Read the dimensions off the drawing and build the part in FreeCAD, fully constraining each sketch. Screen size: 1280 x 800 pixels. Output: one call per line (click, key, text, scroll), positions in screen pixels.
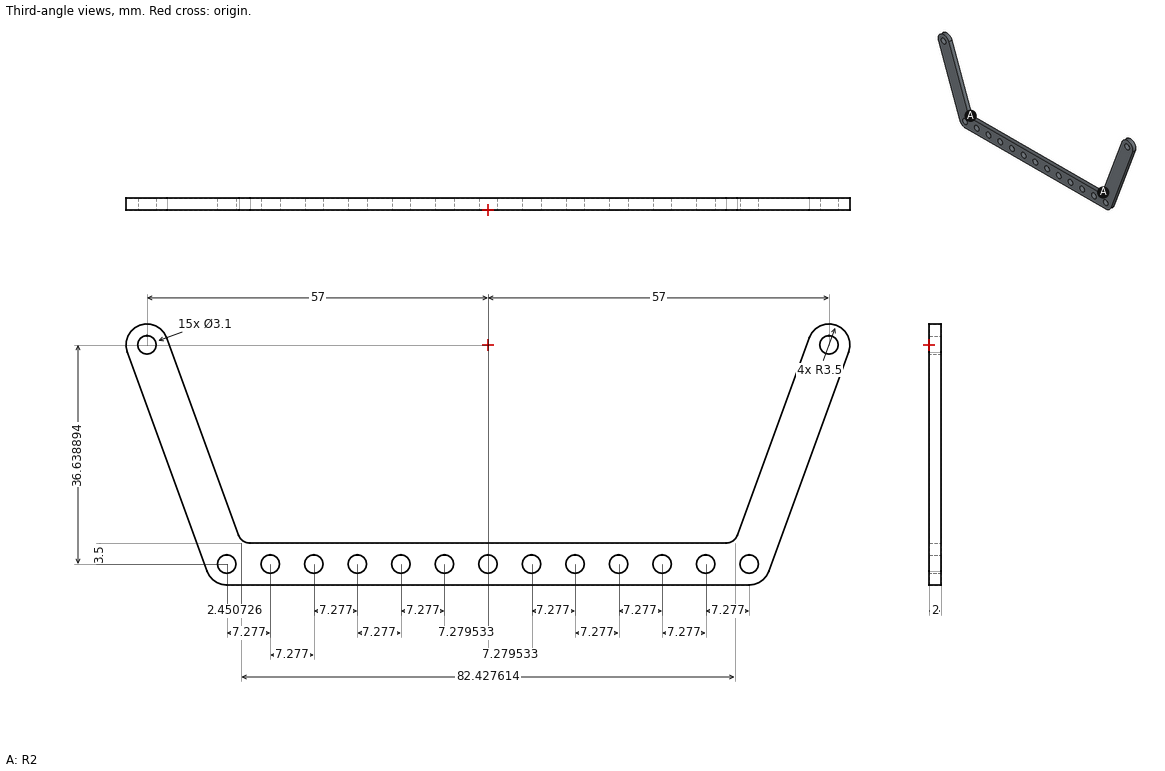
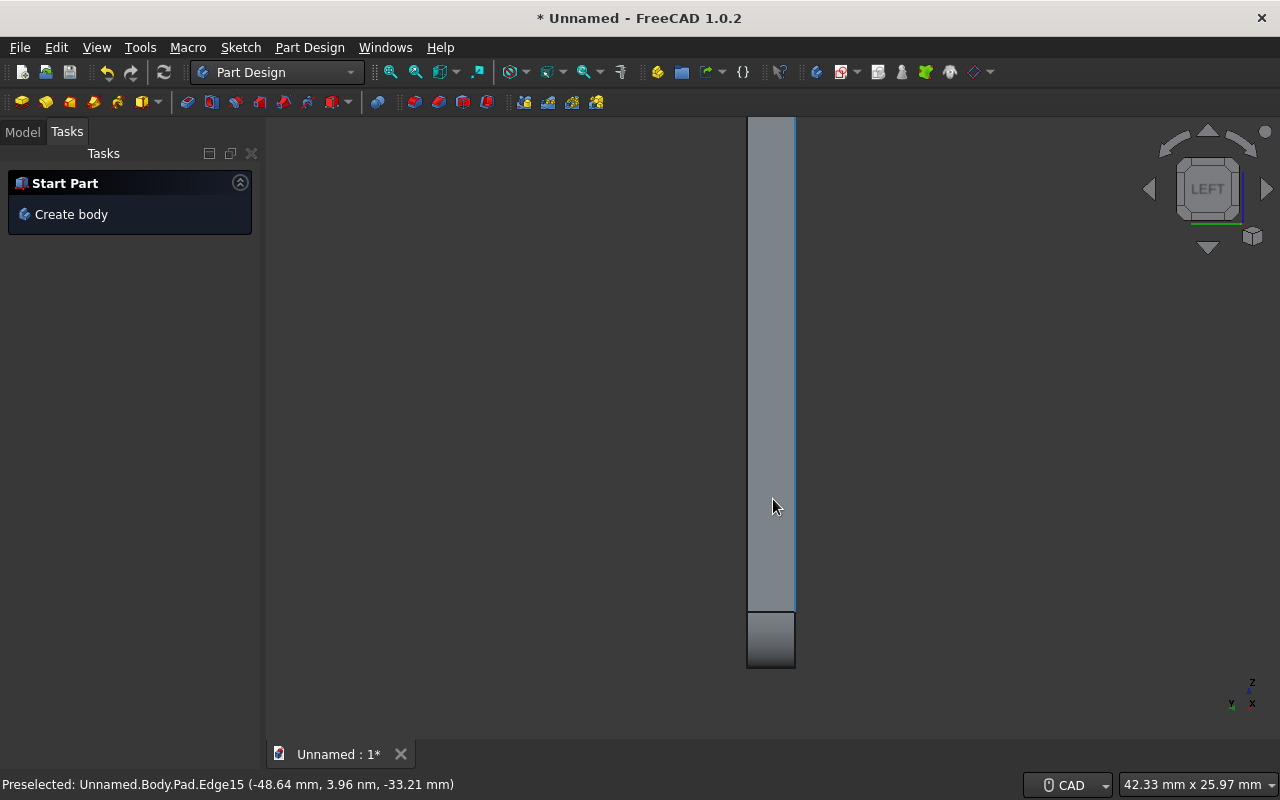
click(392, 72)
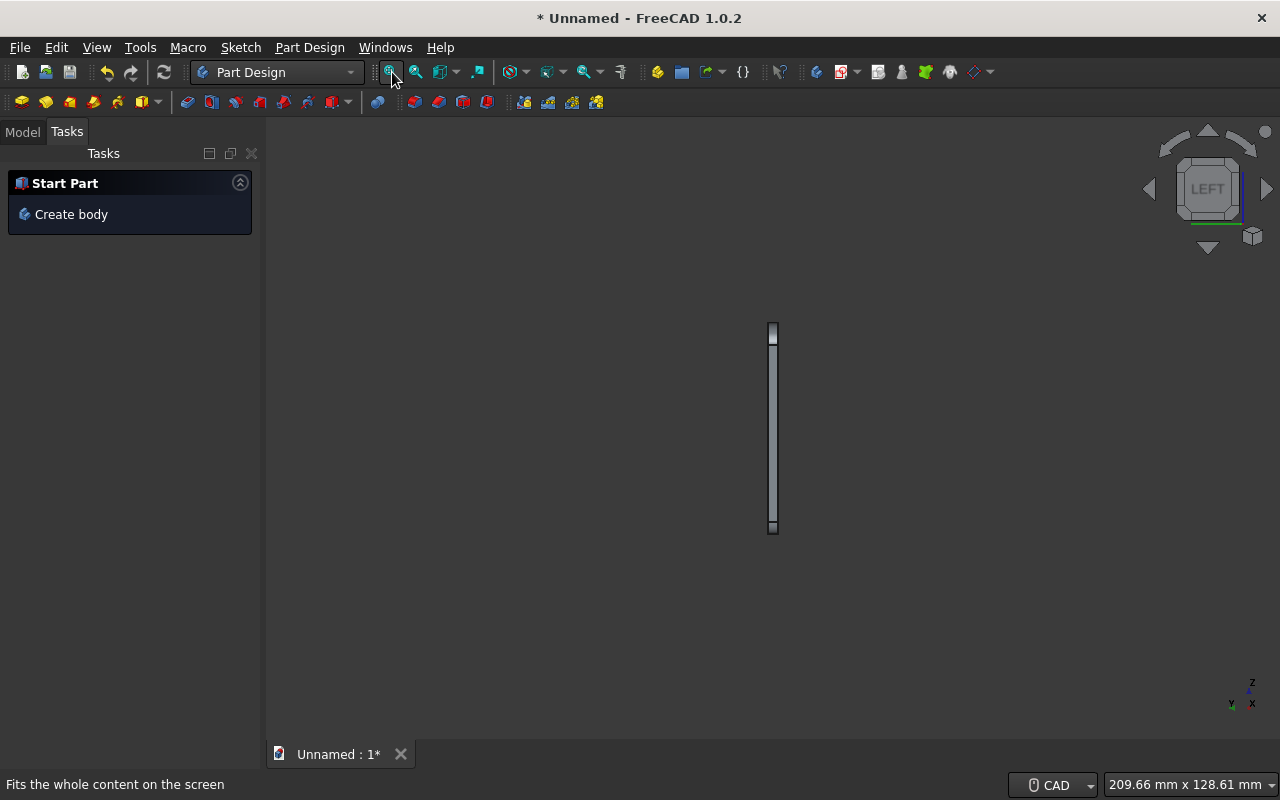
key(v)
key(3)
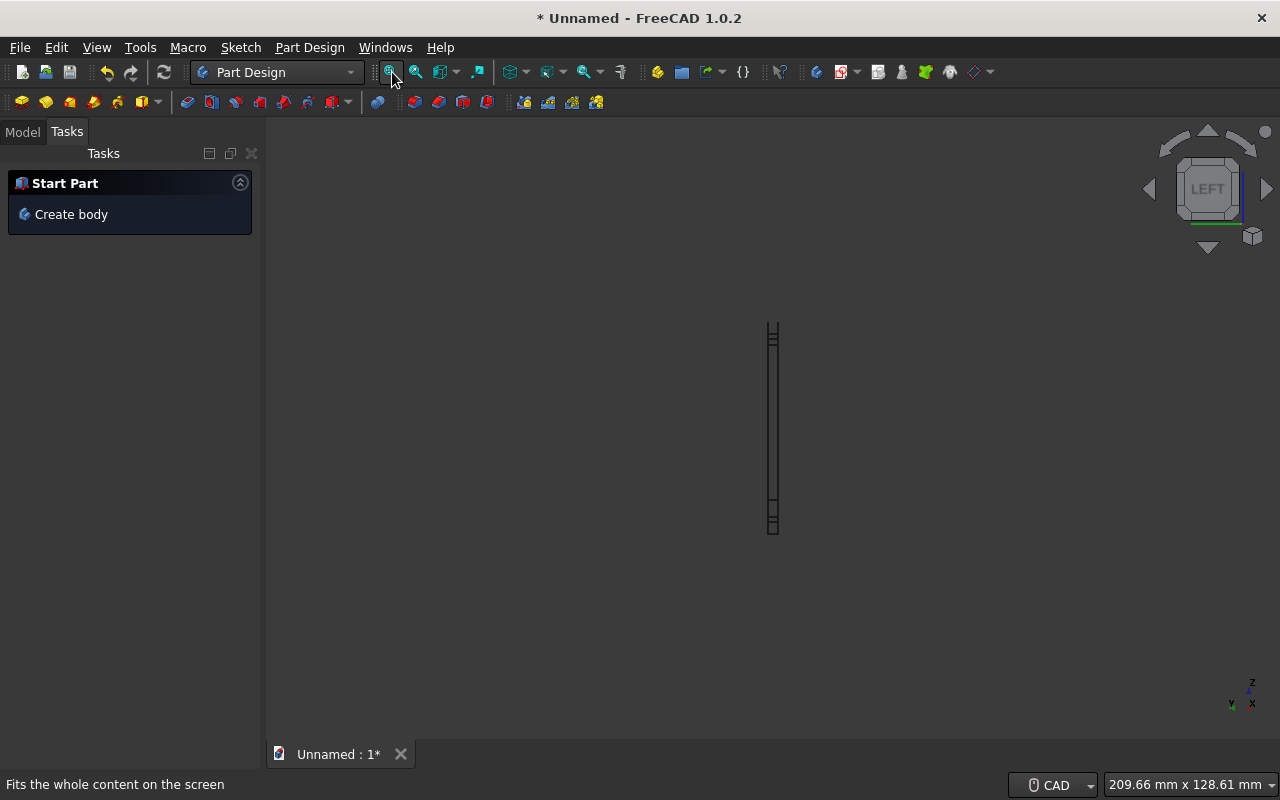
key(0)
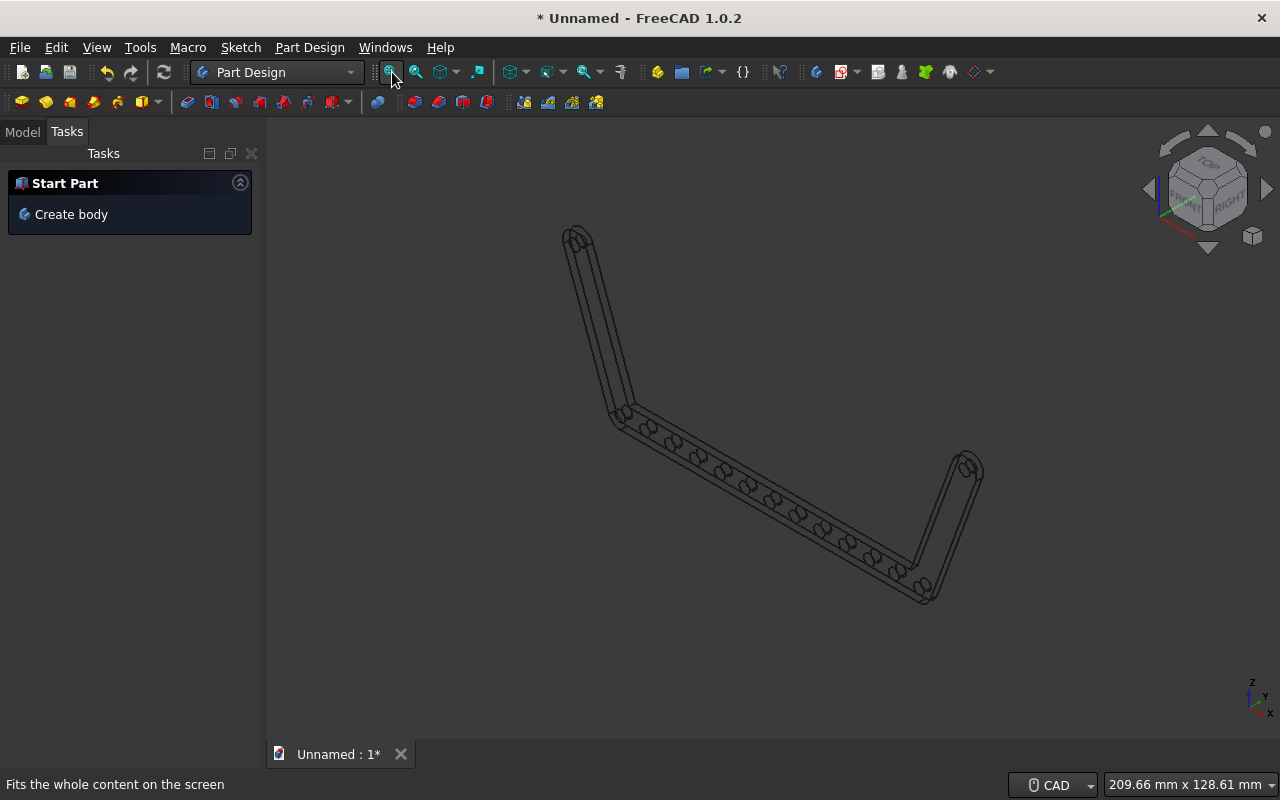
scroll(632, 404, up, 8)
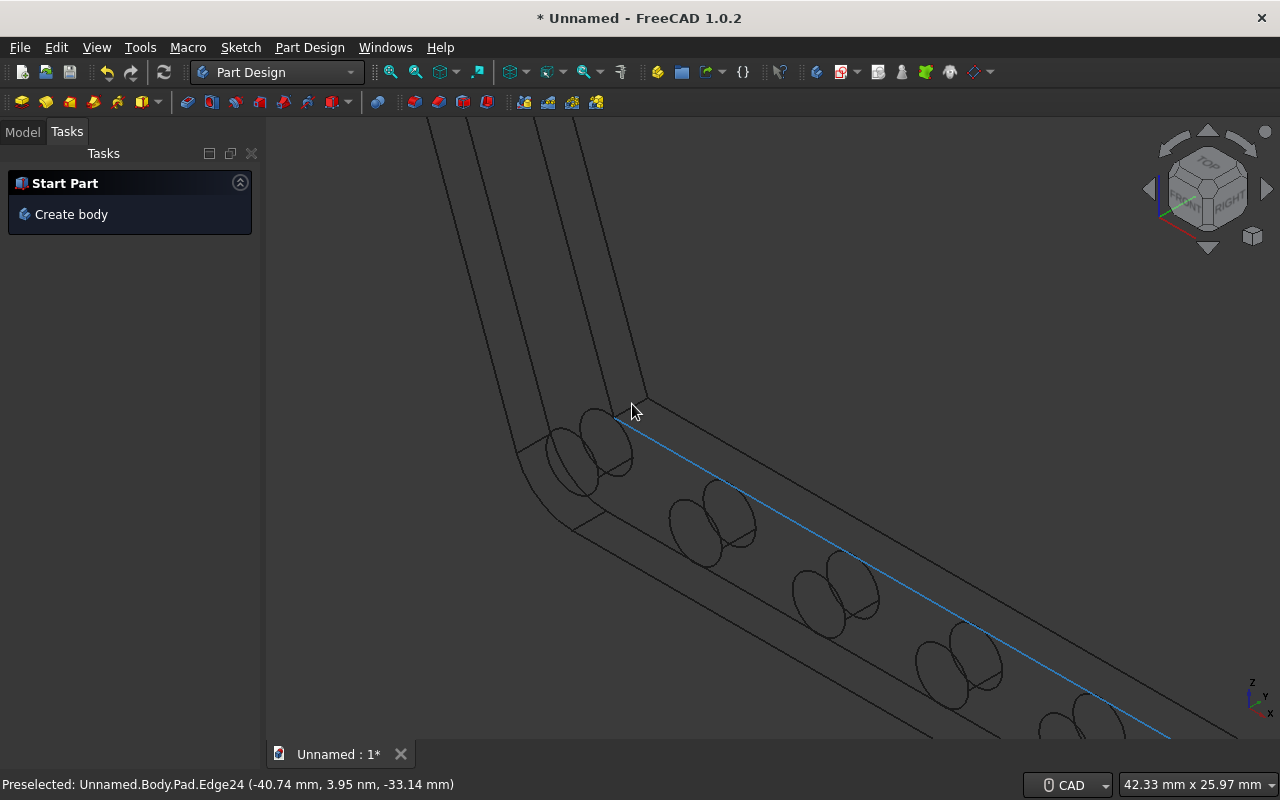
click(631, 407)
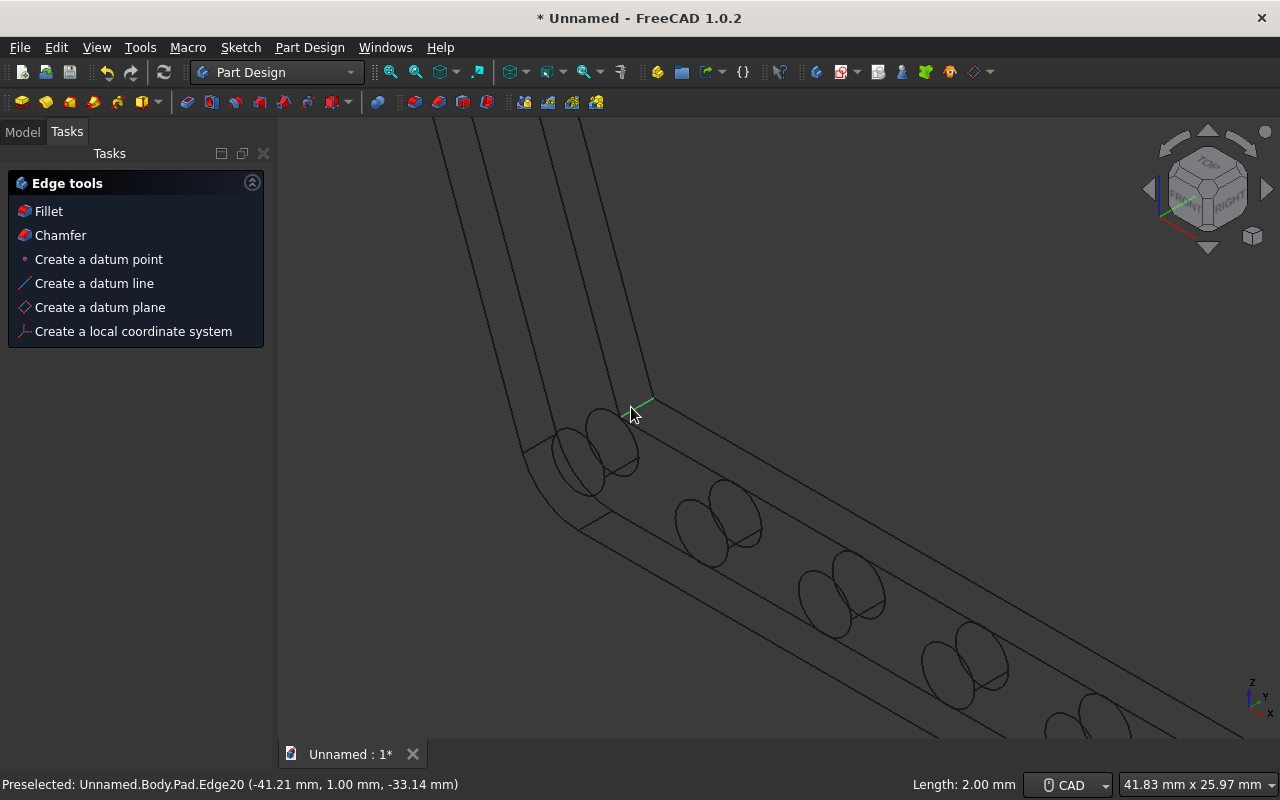
click(392, 72)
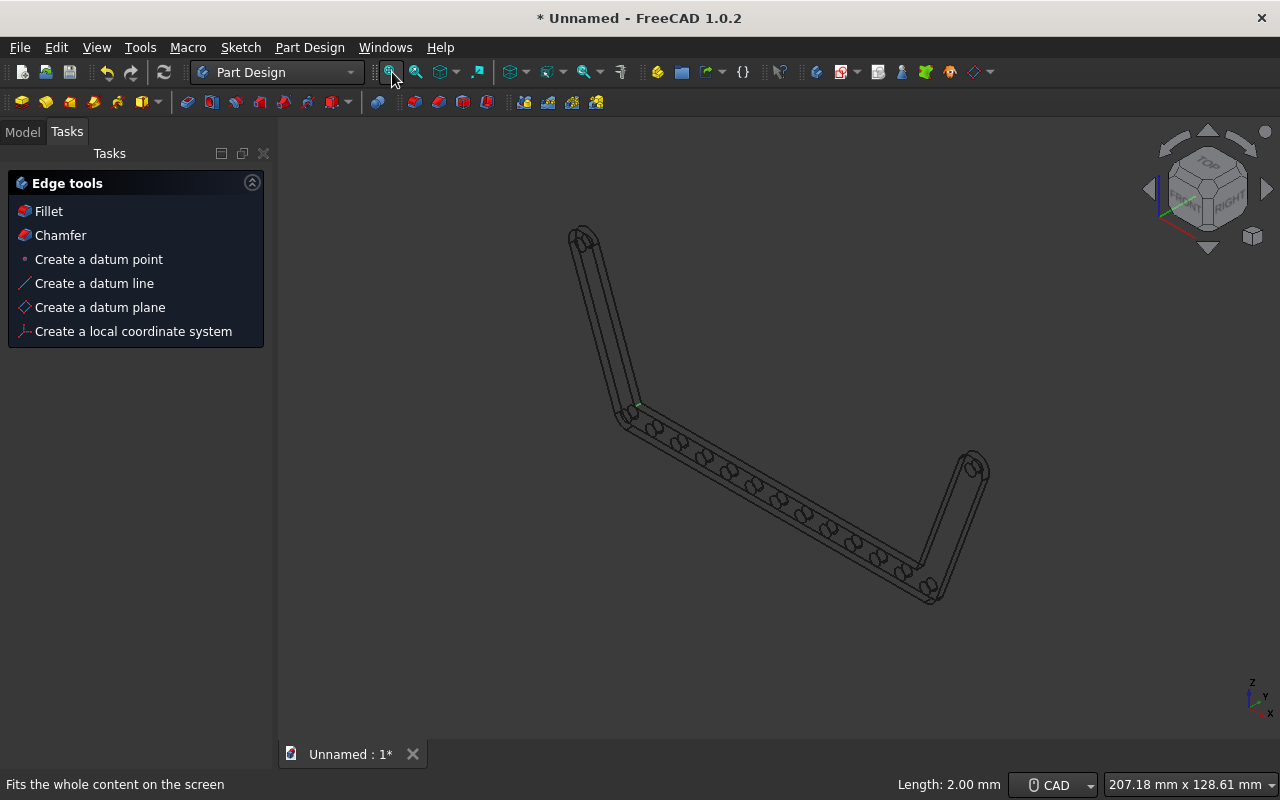
key(2)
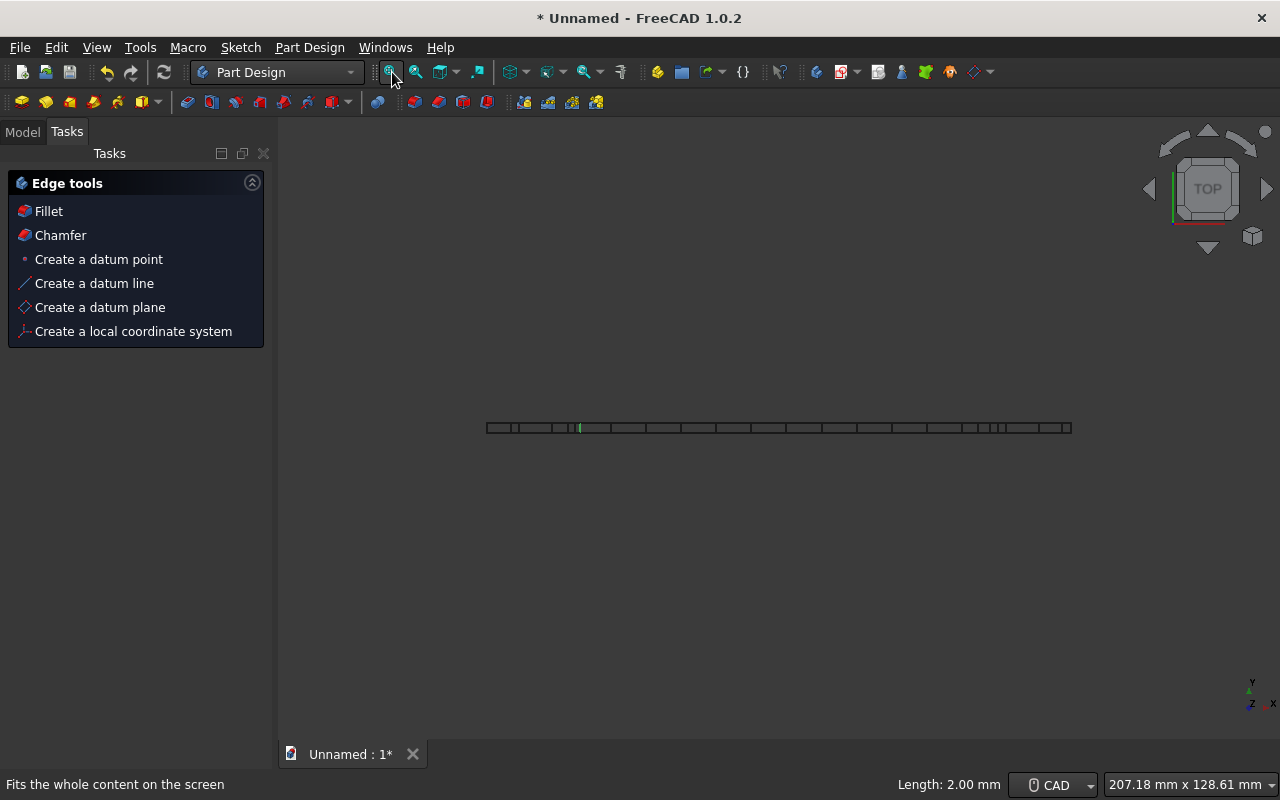
scroll(978, 427, up, 8)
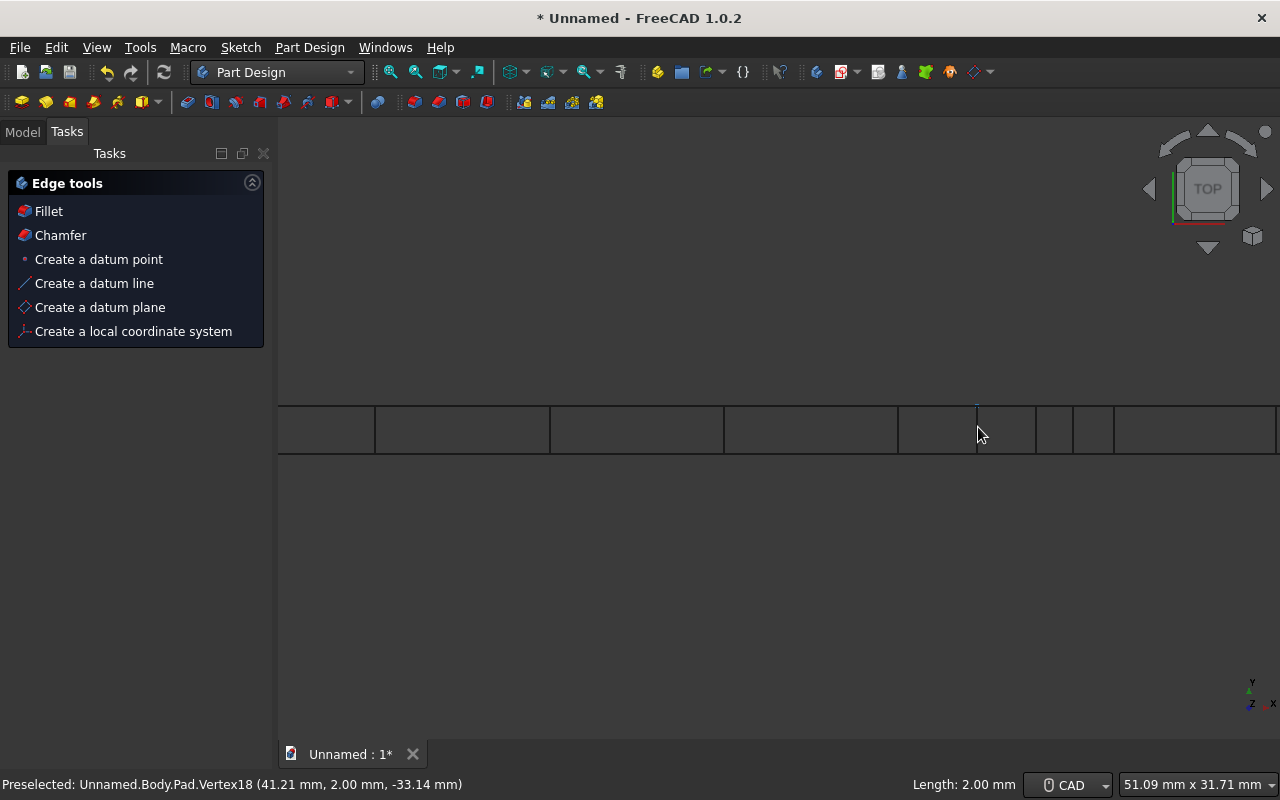
click(977, 429, ctrl)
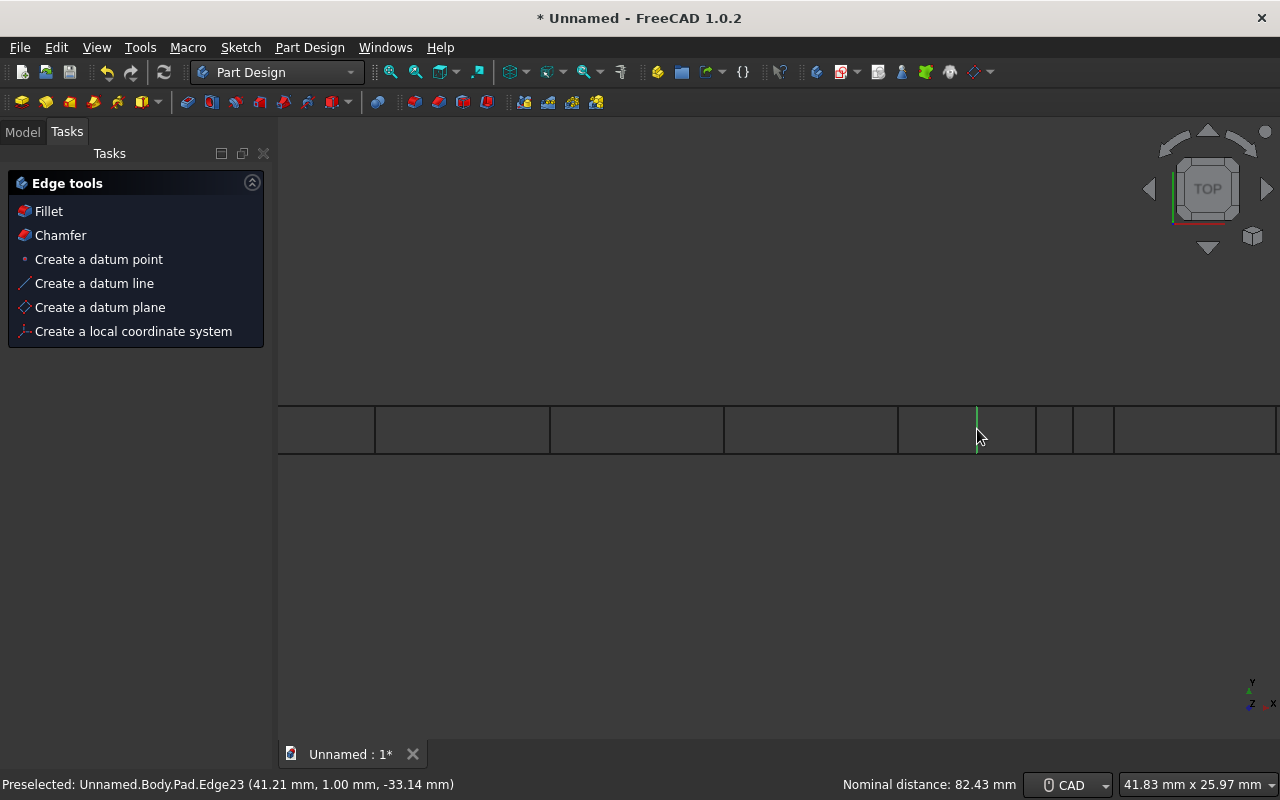
key(v)
key(1)